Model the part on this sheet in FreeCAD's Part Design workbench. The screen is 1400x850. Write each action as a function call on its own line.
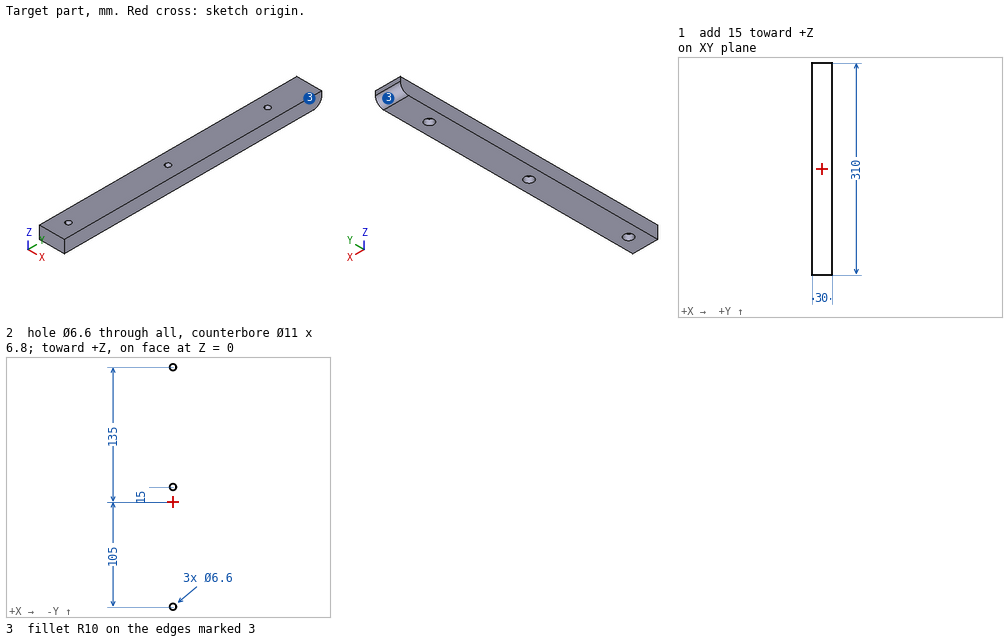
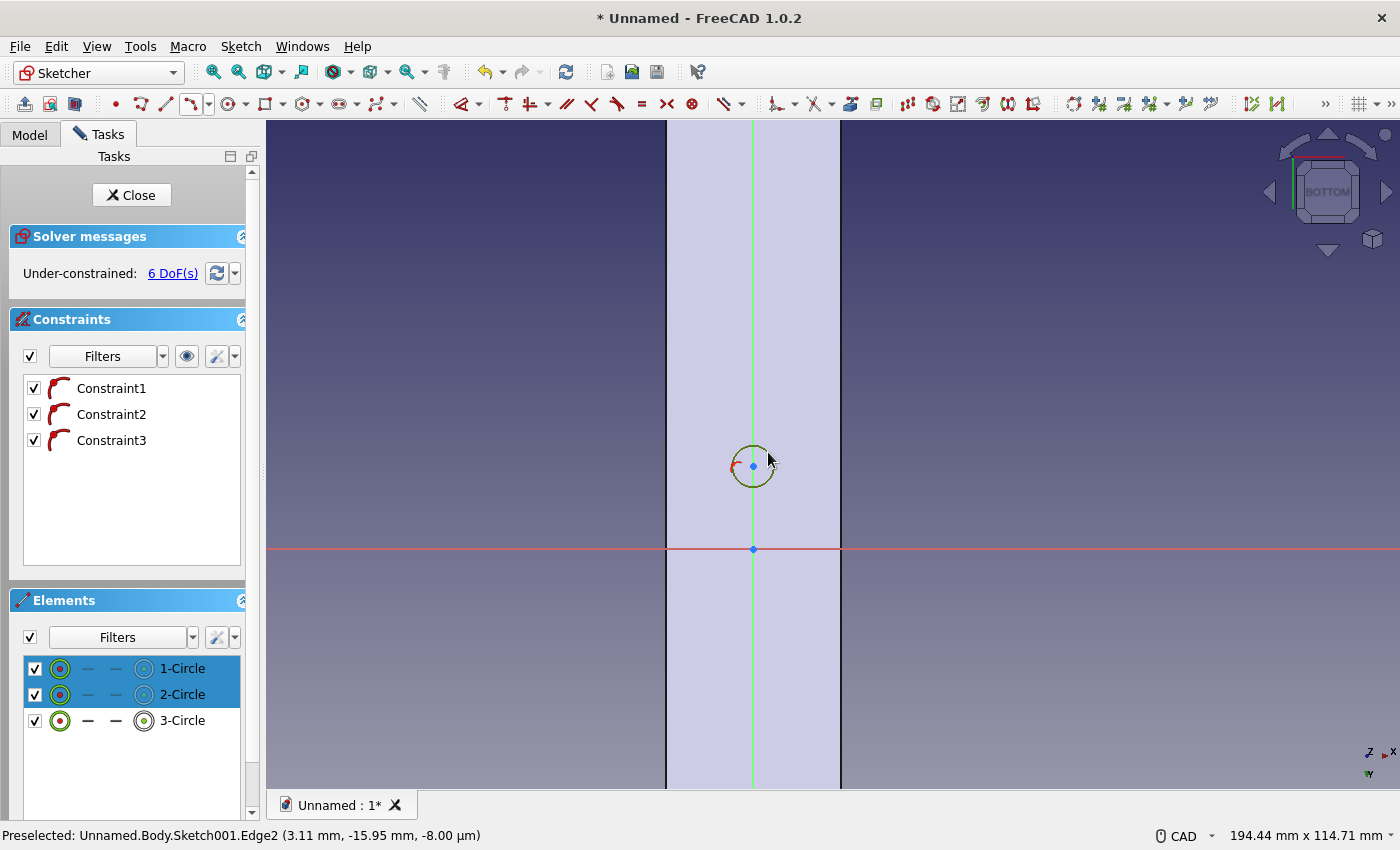
scroll(769, 451, down, 6)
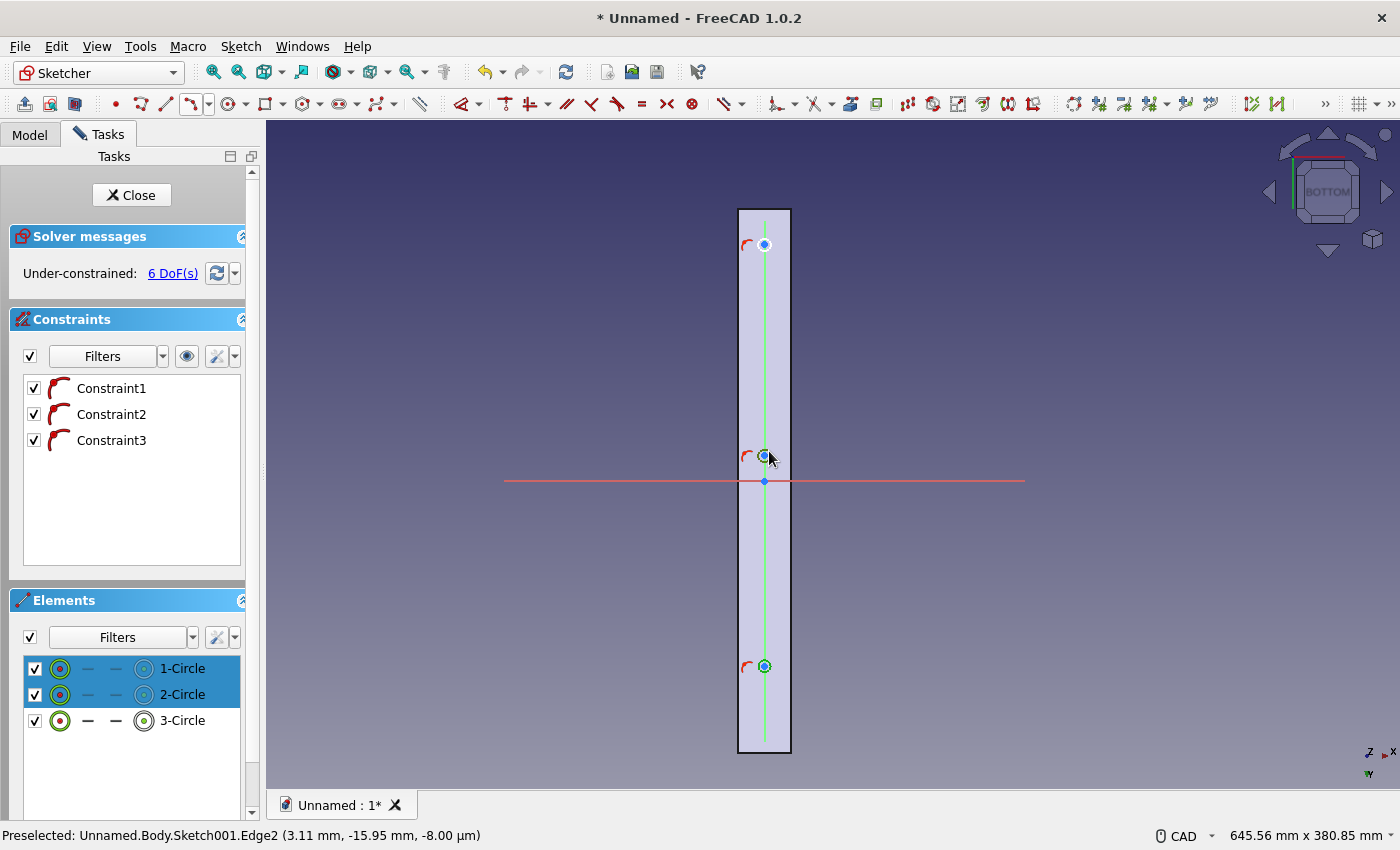
scroll(769, 241, up, 6)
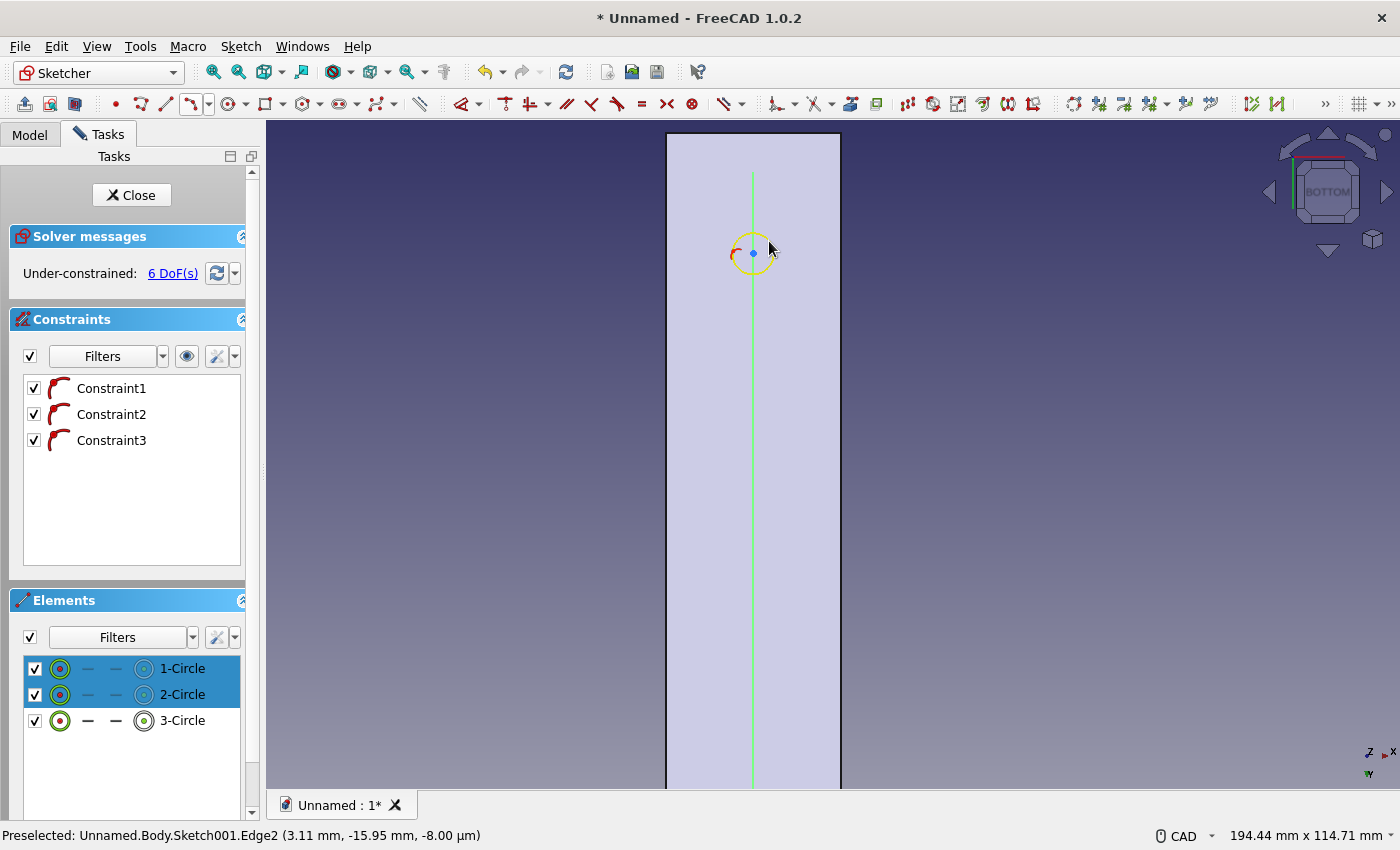
click(768, 239)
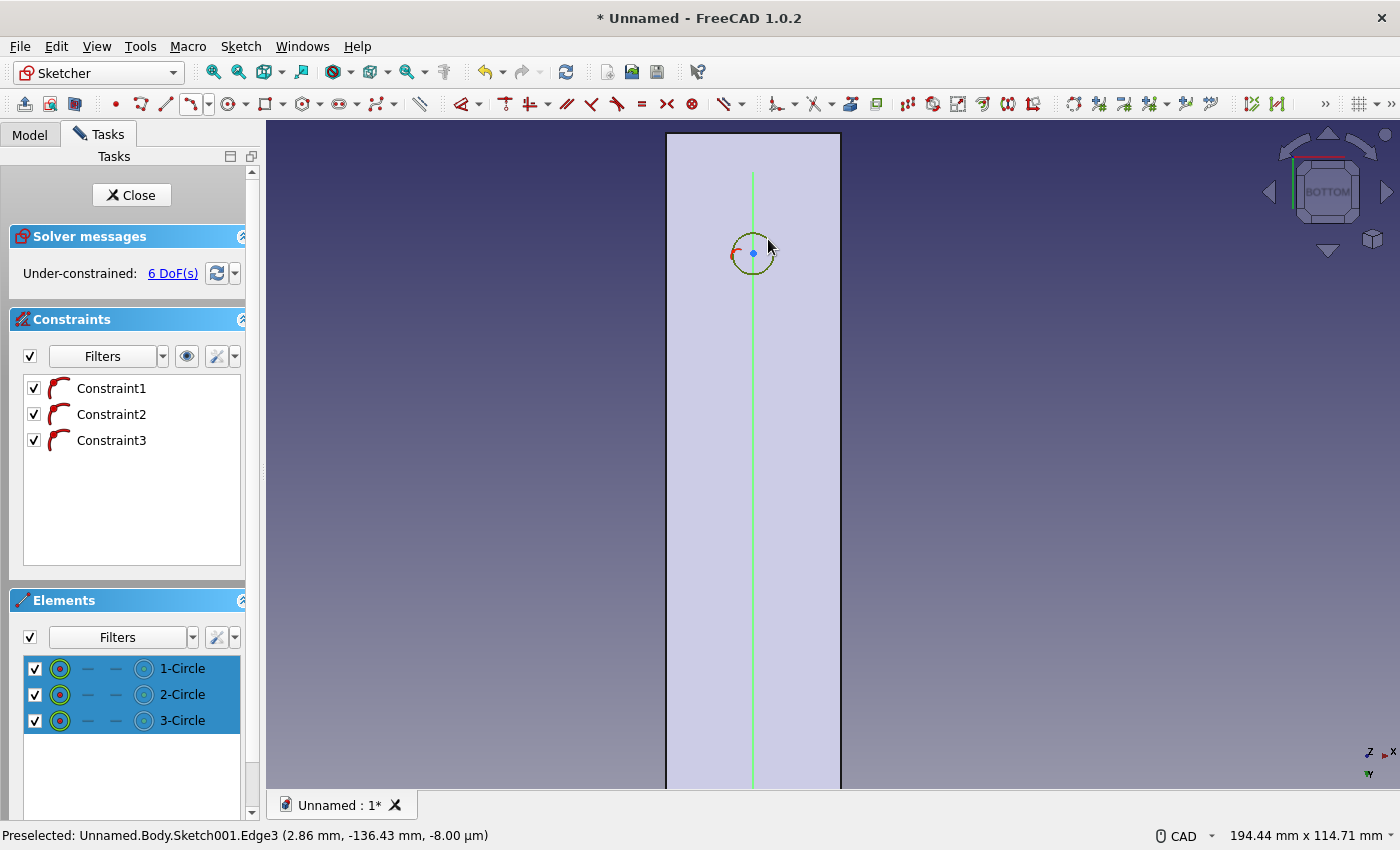
key(e)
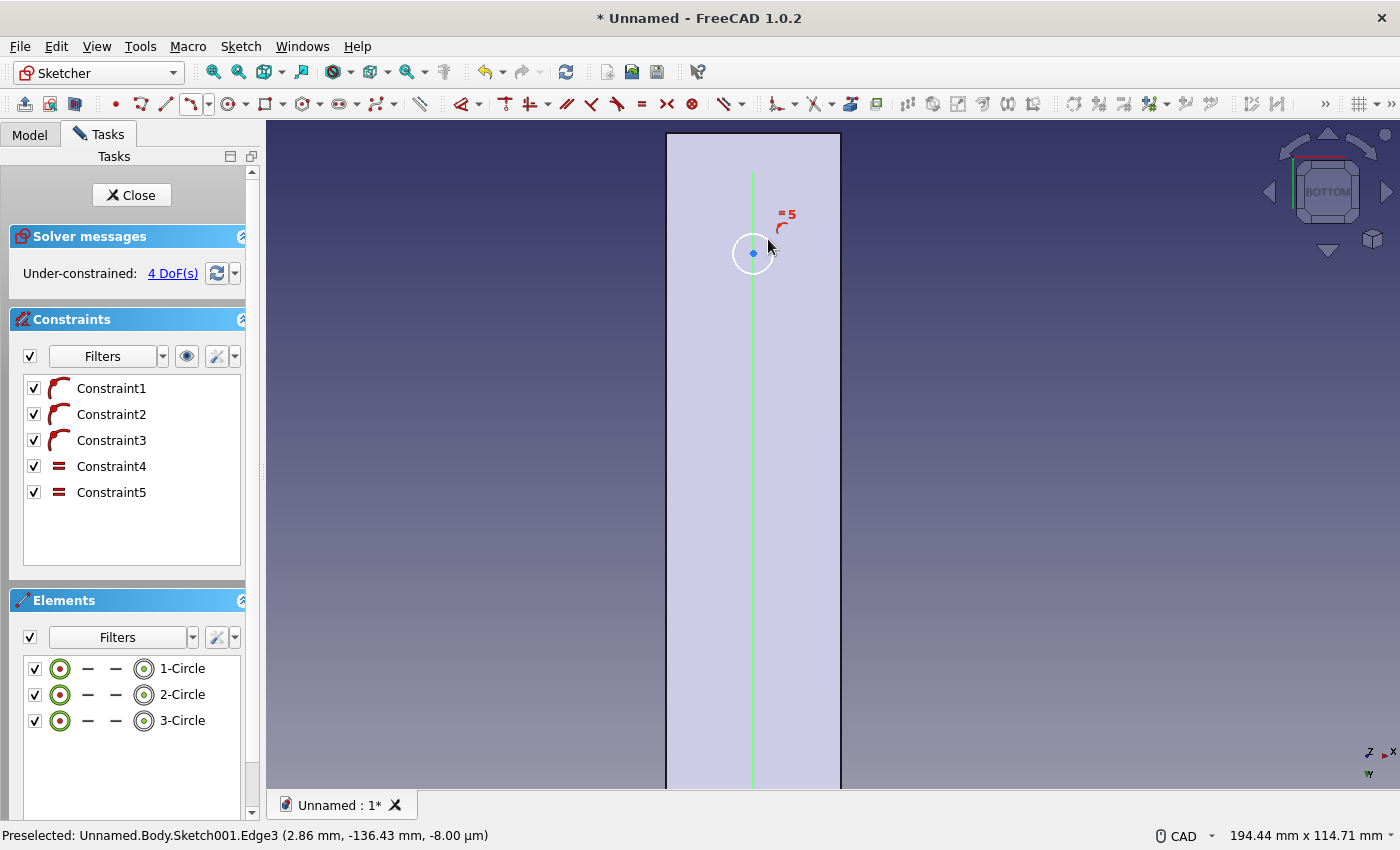
click(460, 104)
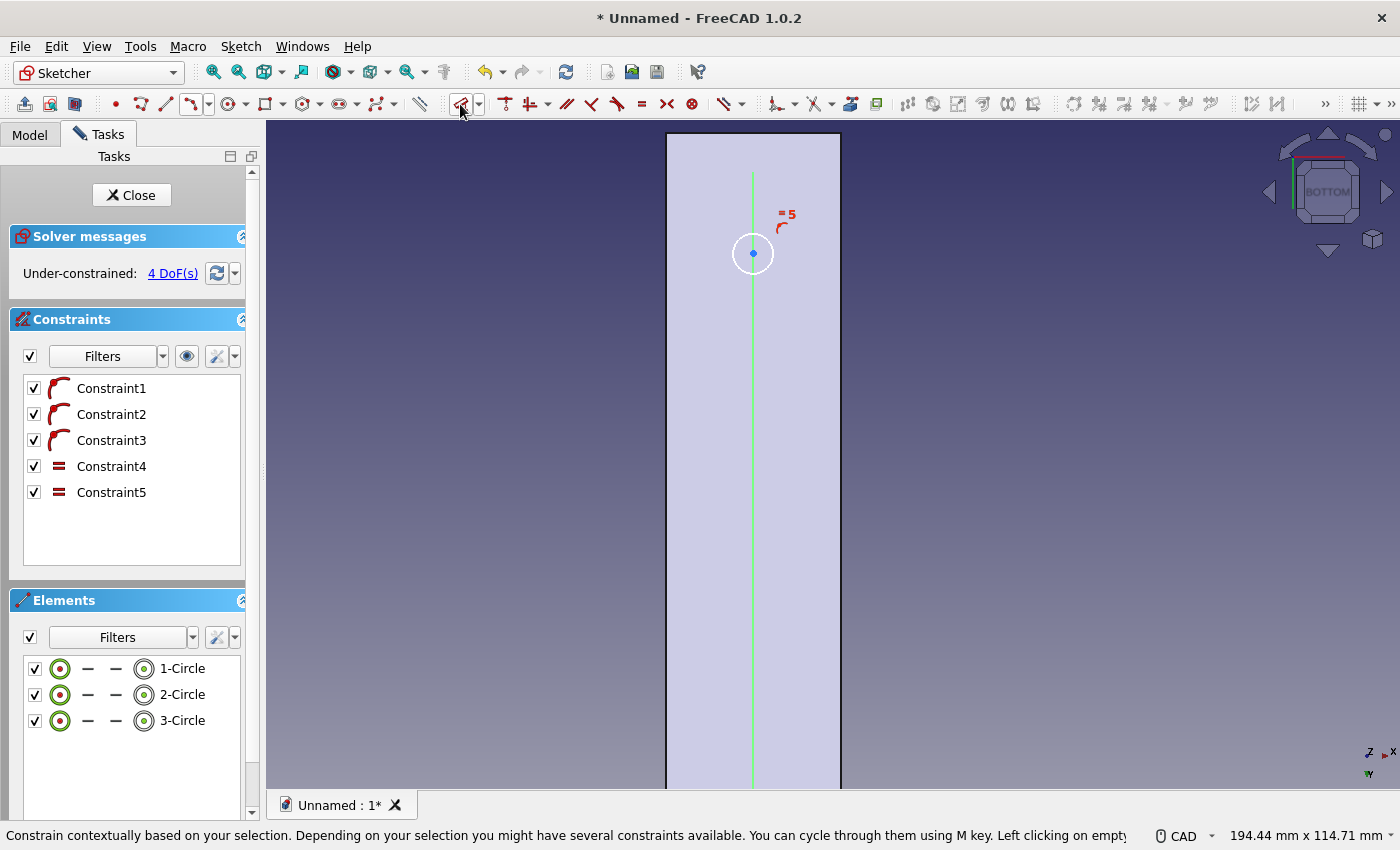
scroll(769, 241, down, 6)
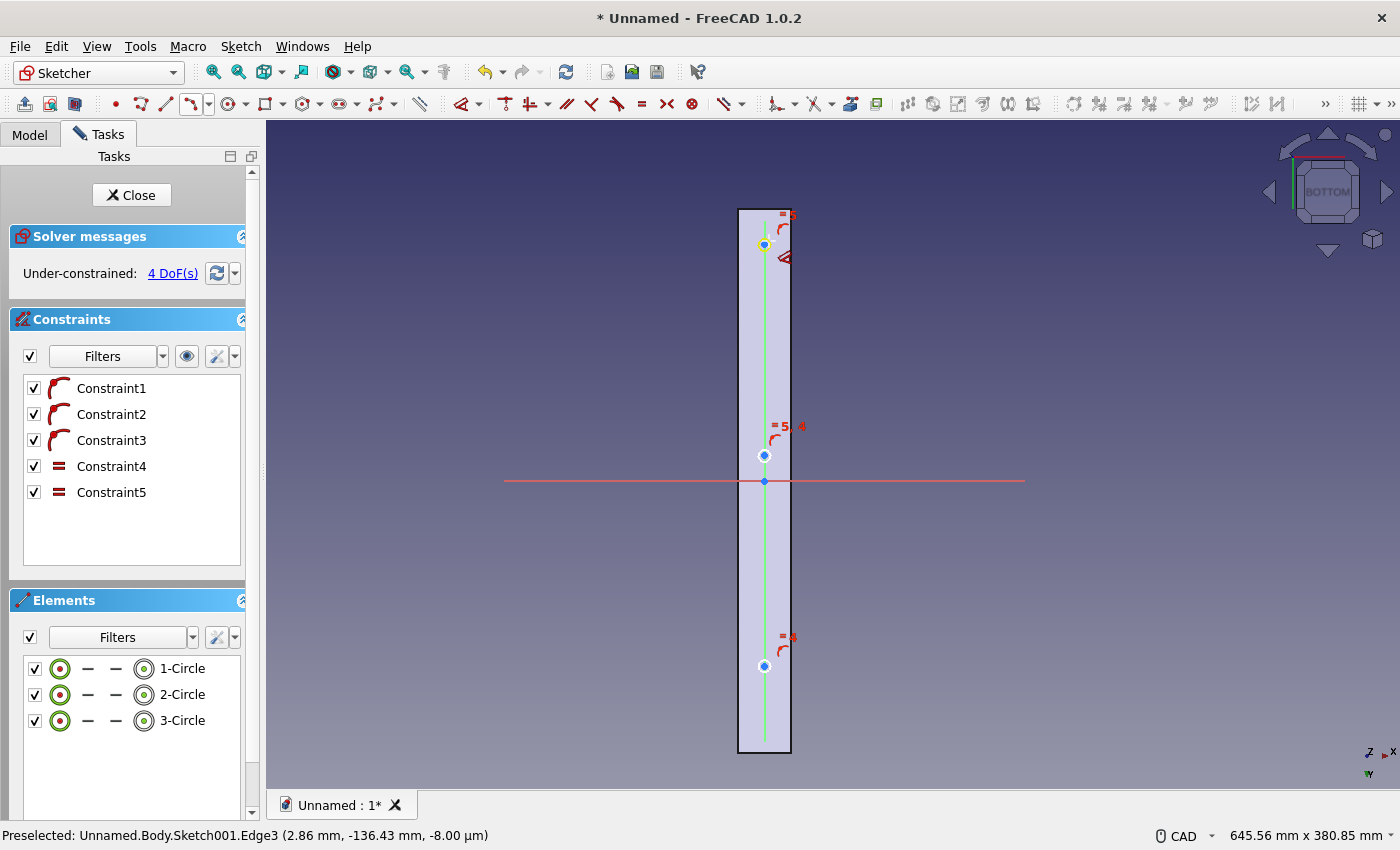
scroll(769, 662, up, 7)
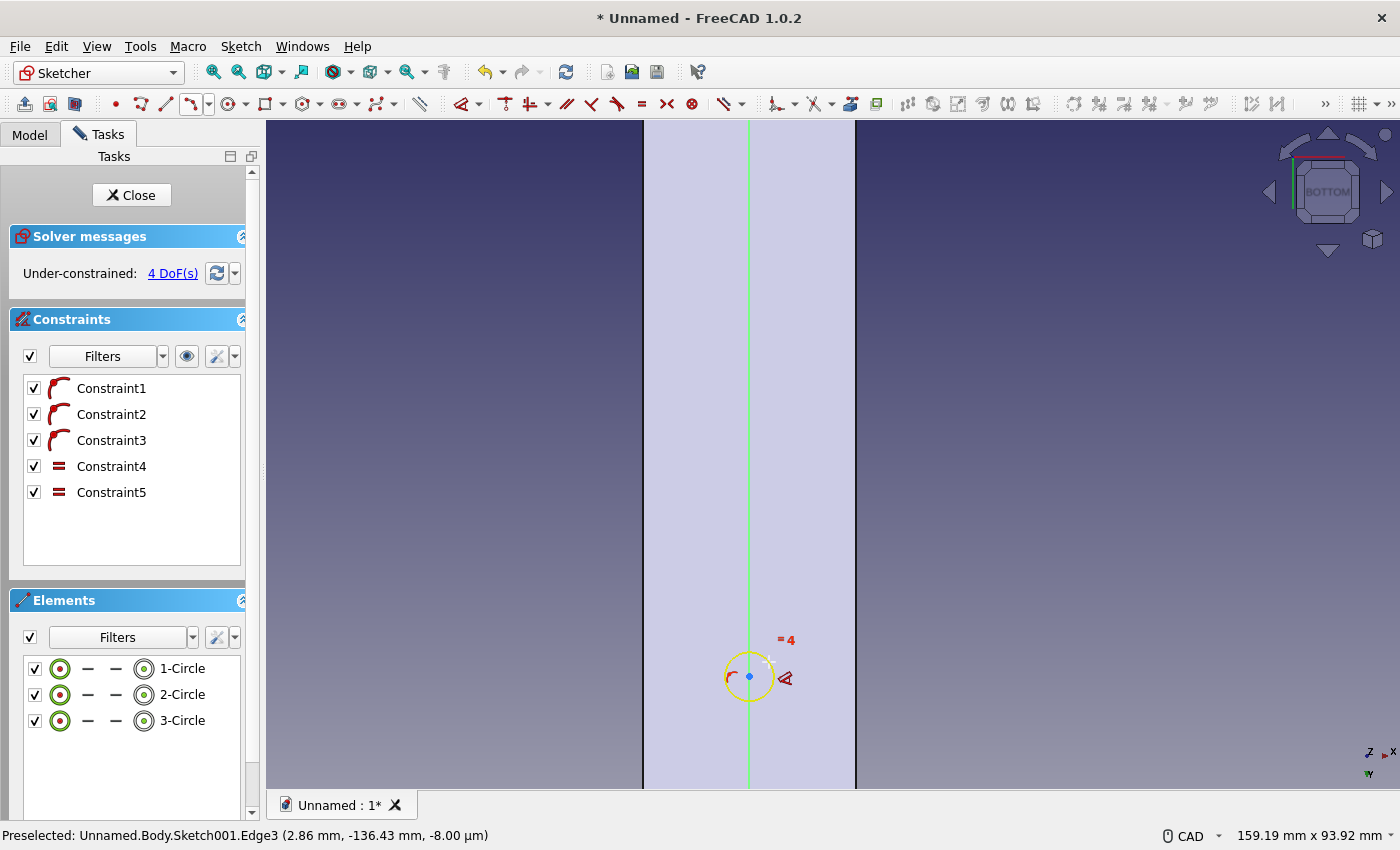
click(767, 659)
click(790, 636)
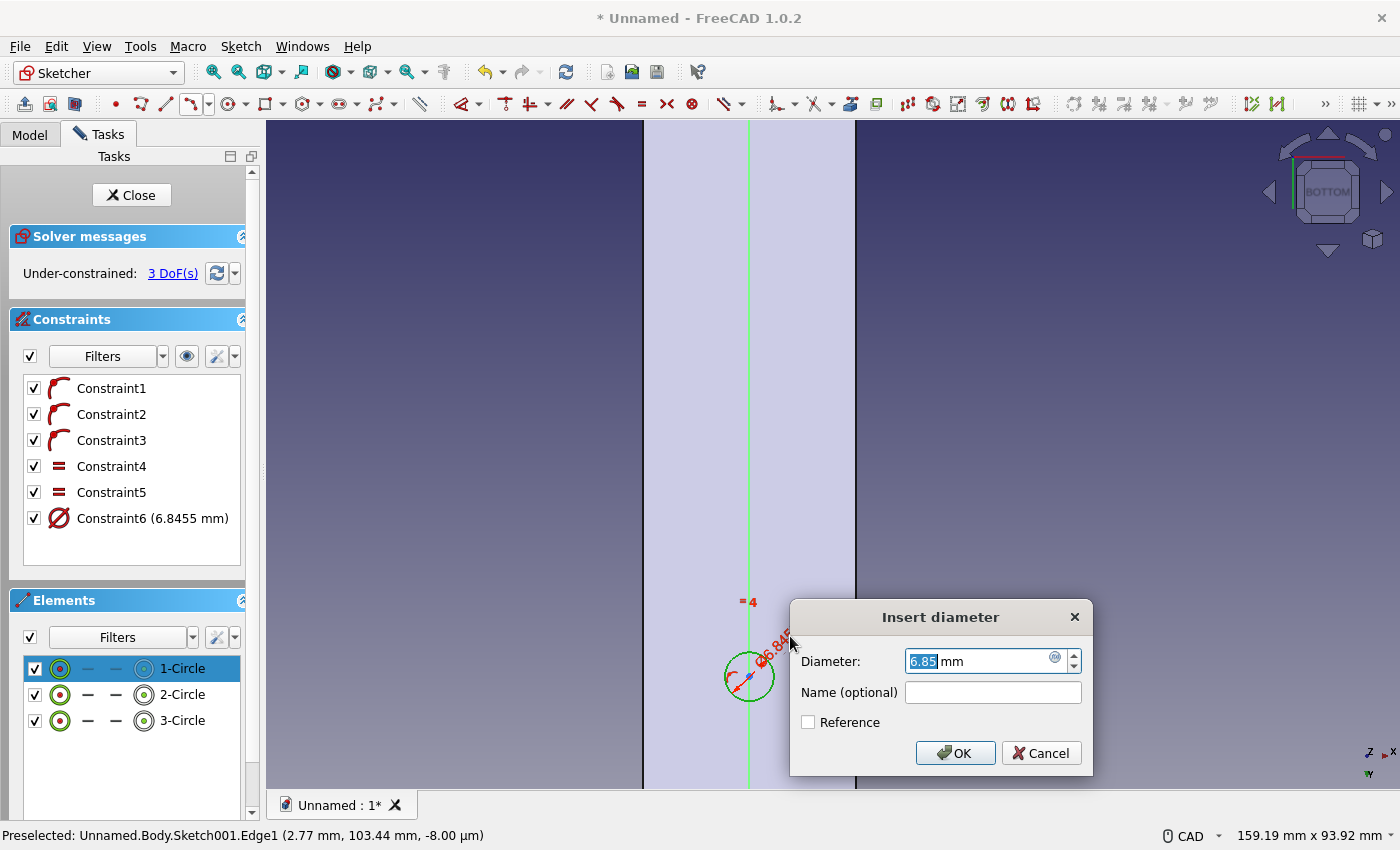
text(6.6)
key(Return)